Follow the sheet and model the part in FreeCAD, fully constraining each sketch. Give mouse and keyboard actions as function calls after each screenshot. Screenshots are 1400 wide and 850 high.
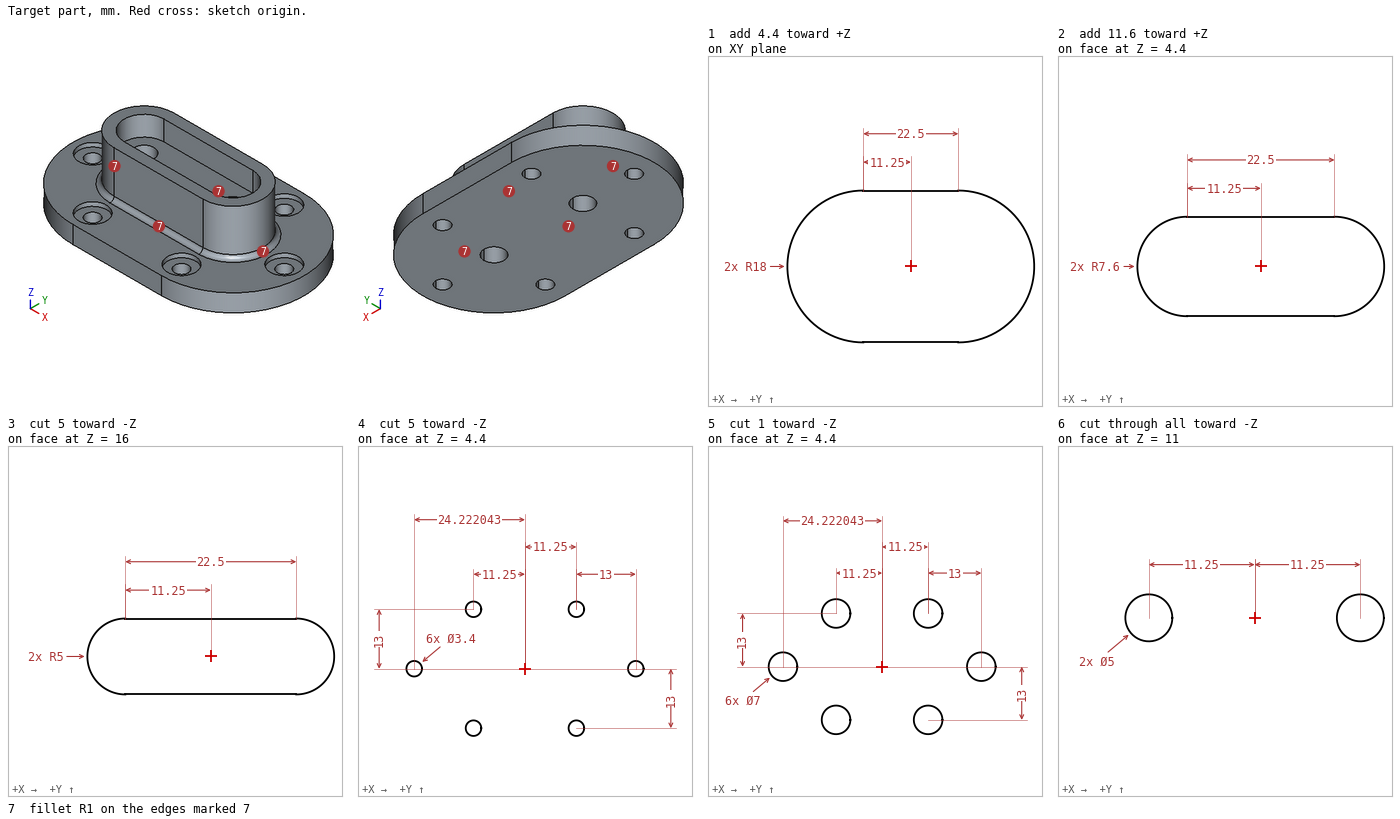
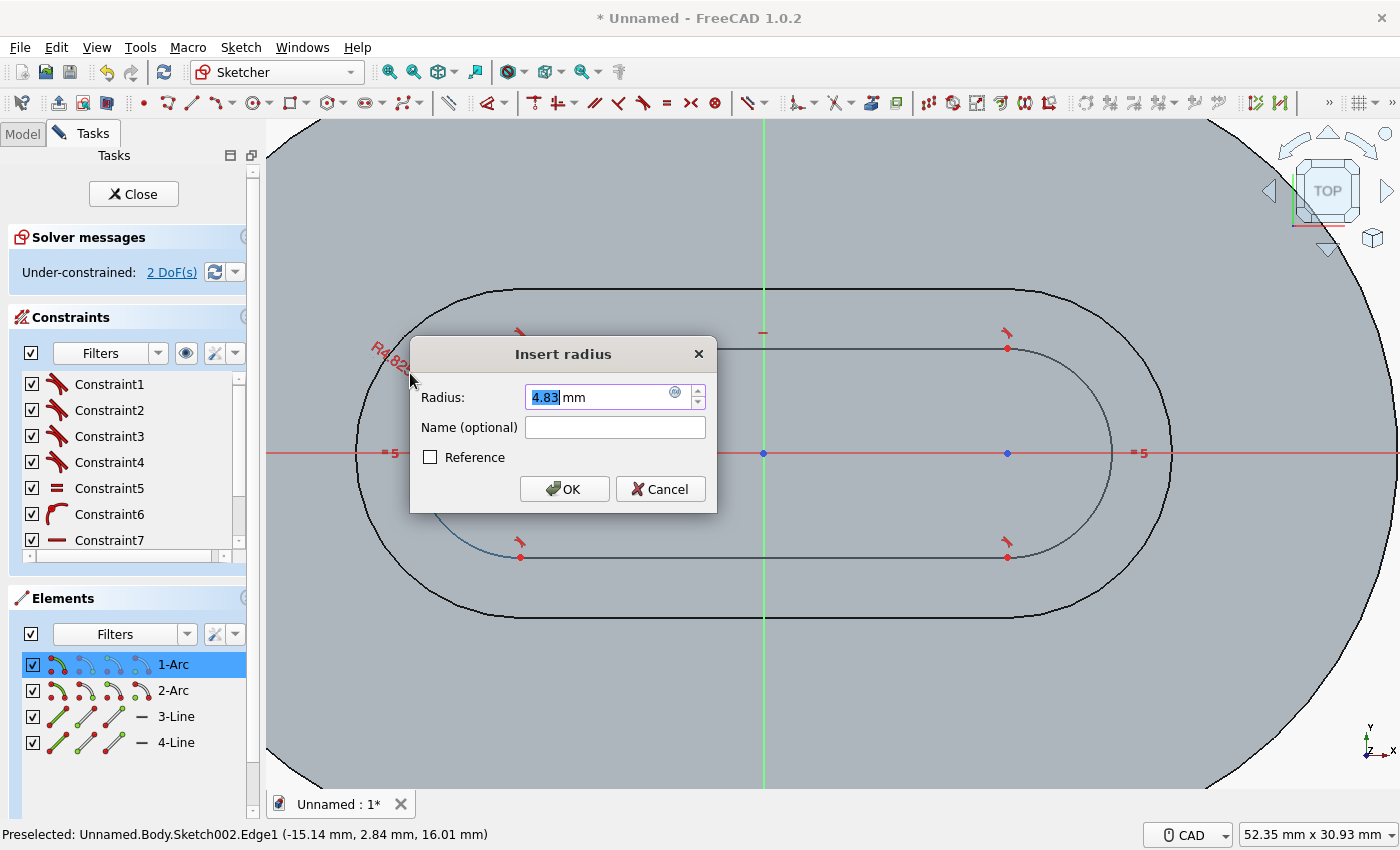
text(5)
key(Return)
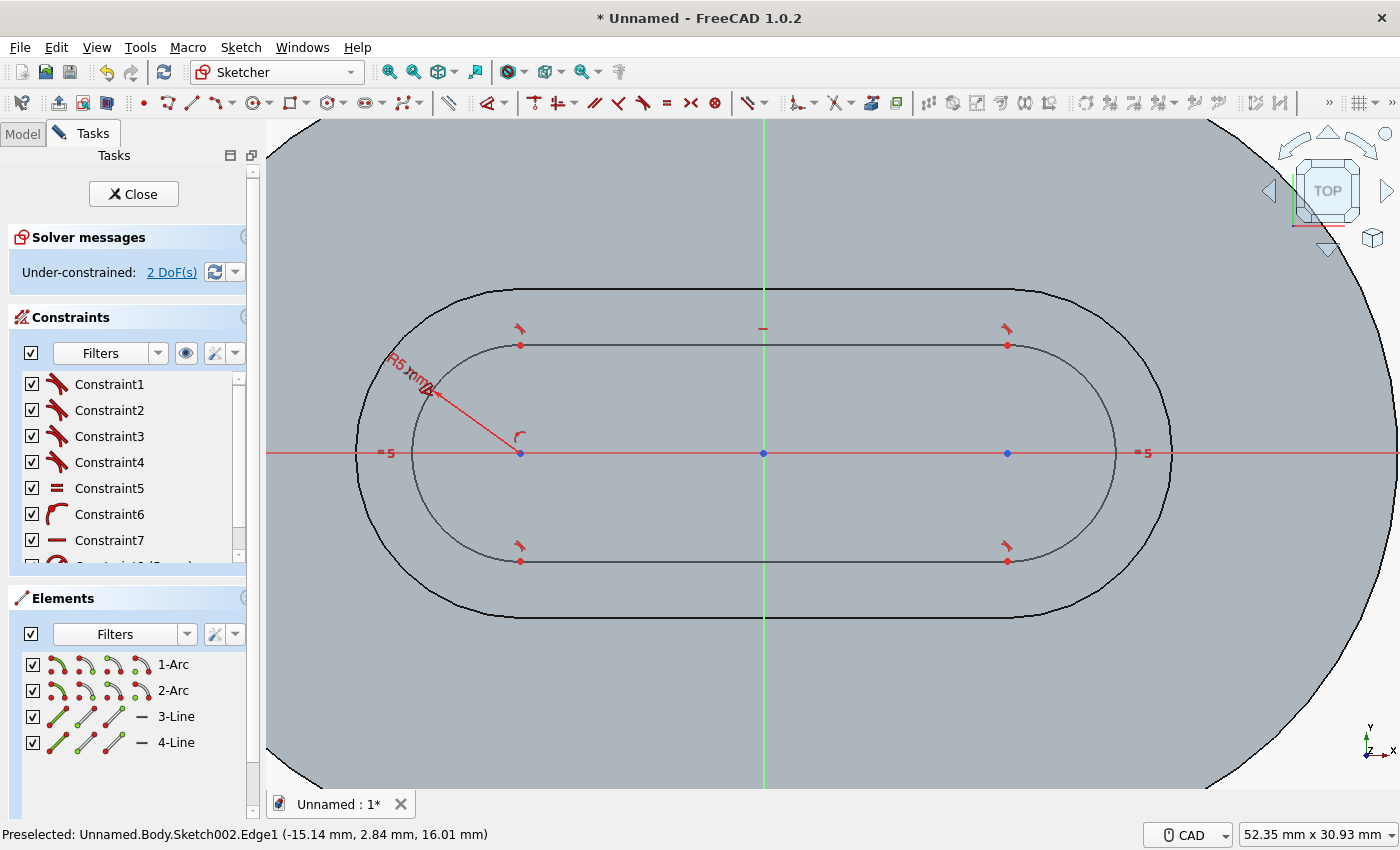
click(667, 345)
click(652, 311)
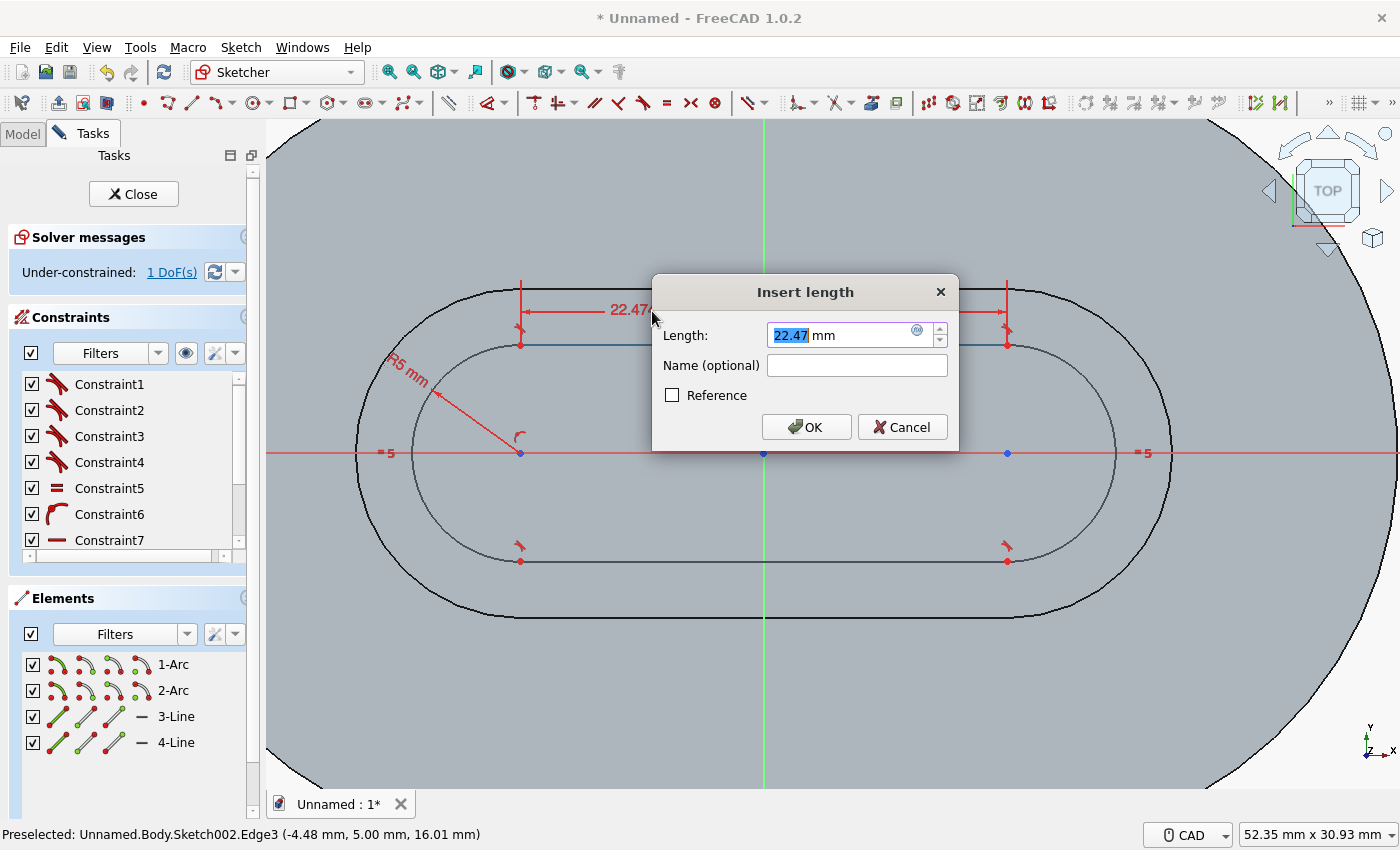
text(22.5)
key(Return)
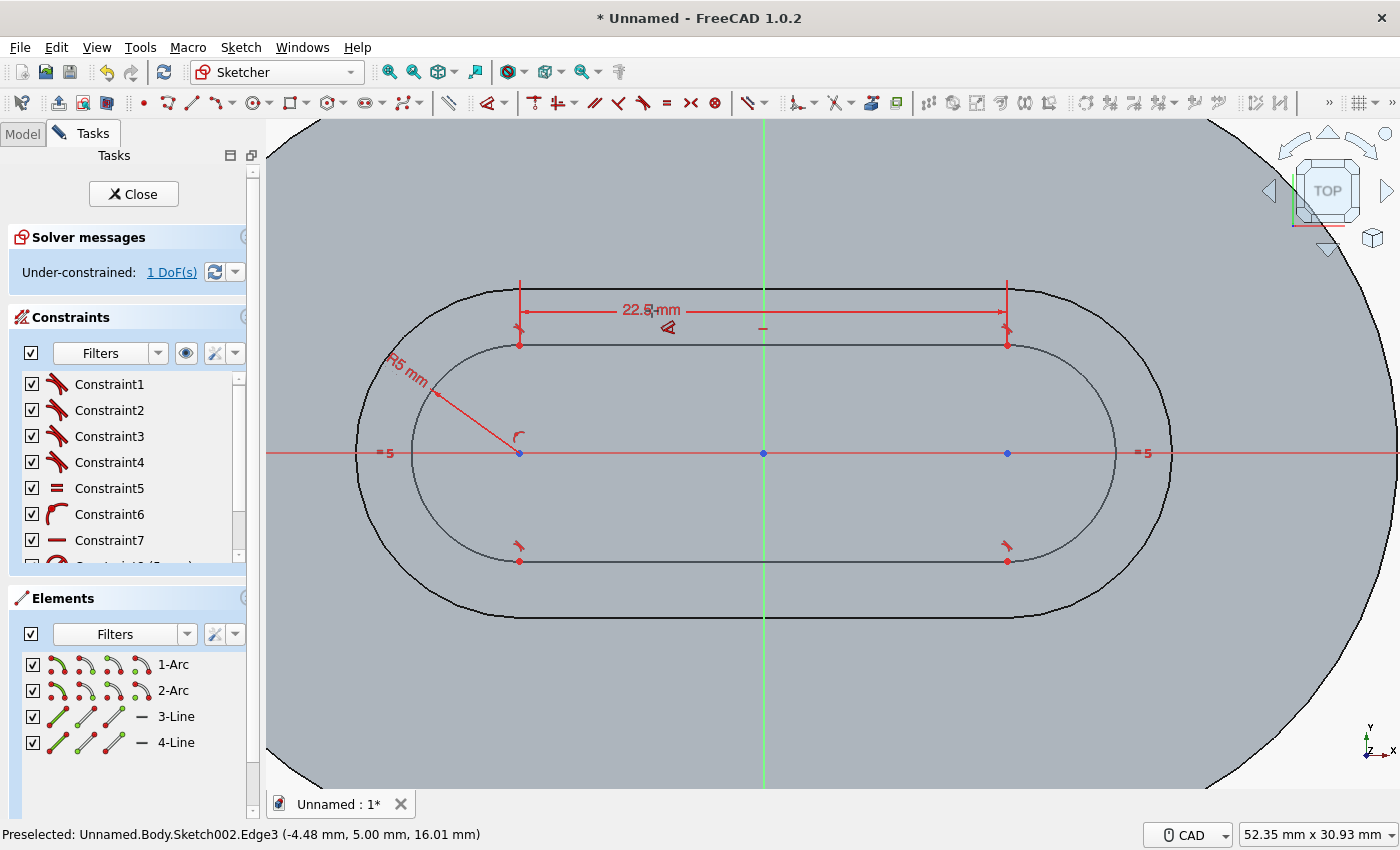
click(520, 345)
click(557, 311)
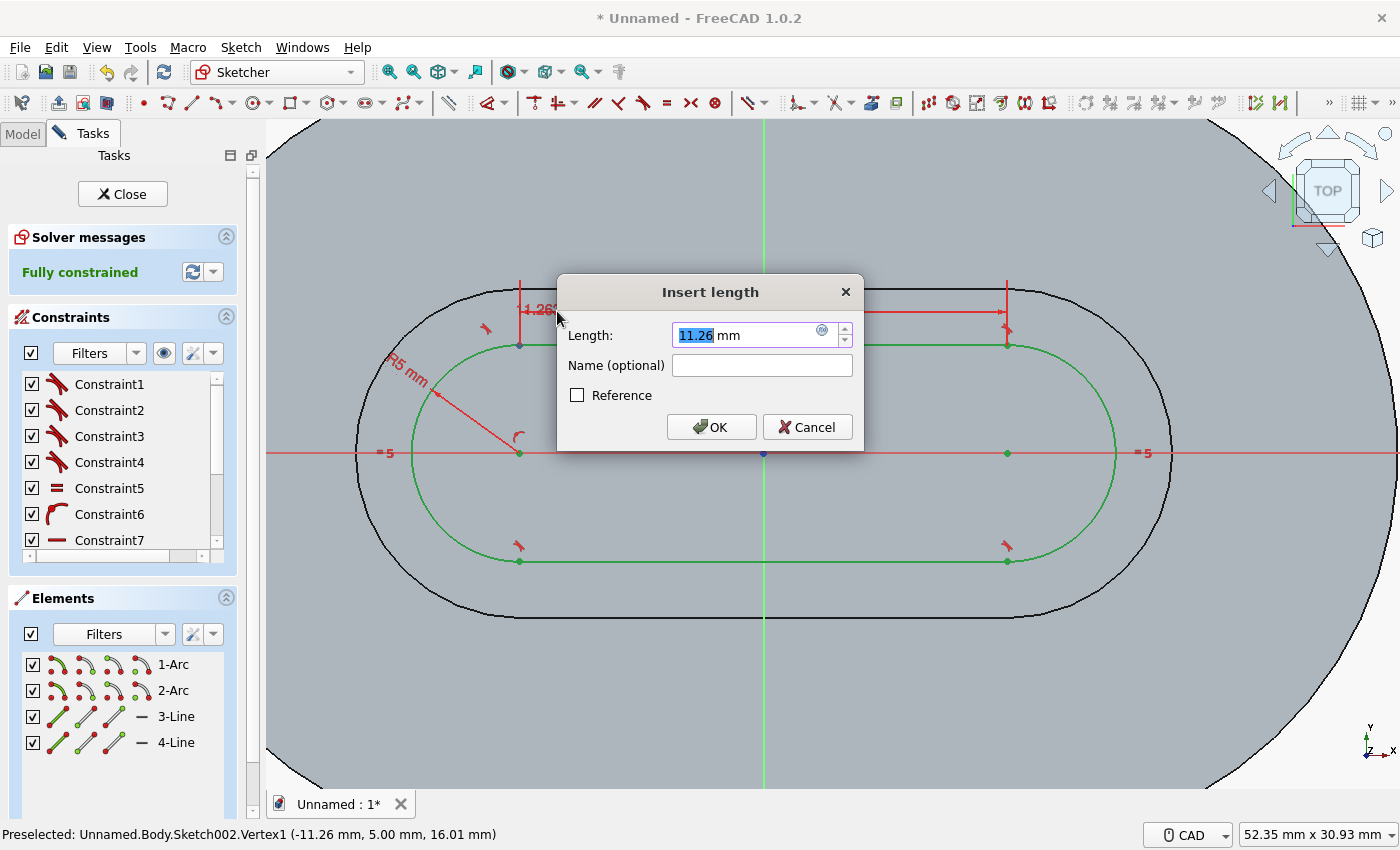
text(11.25)
key(Return)
key(Escape)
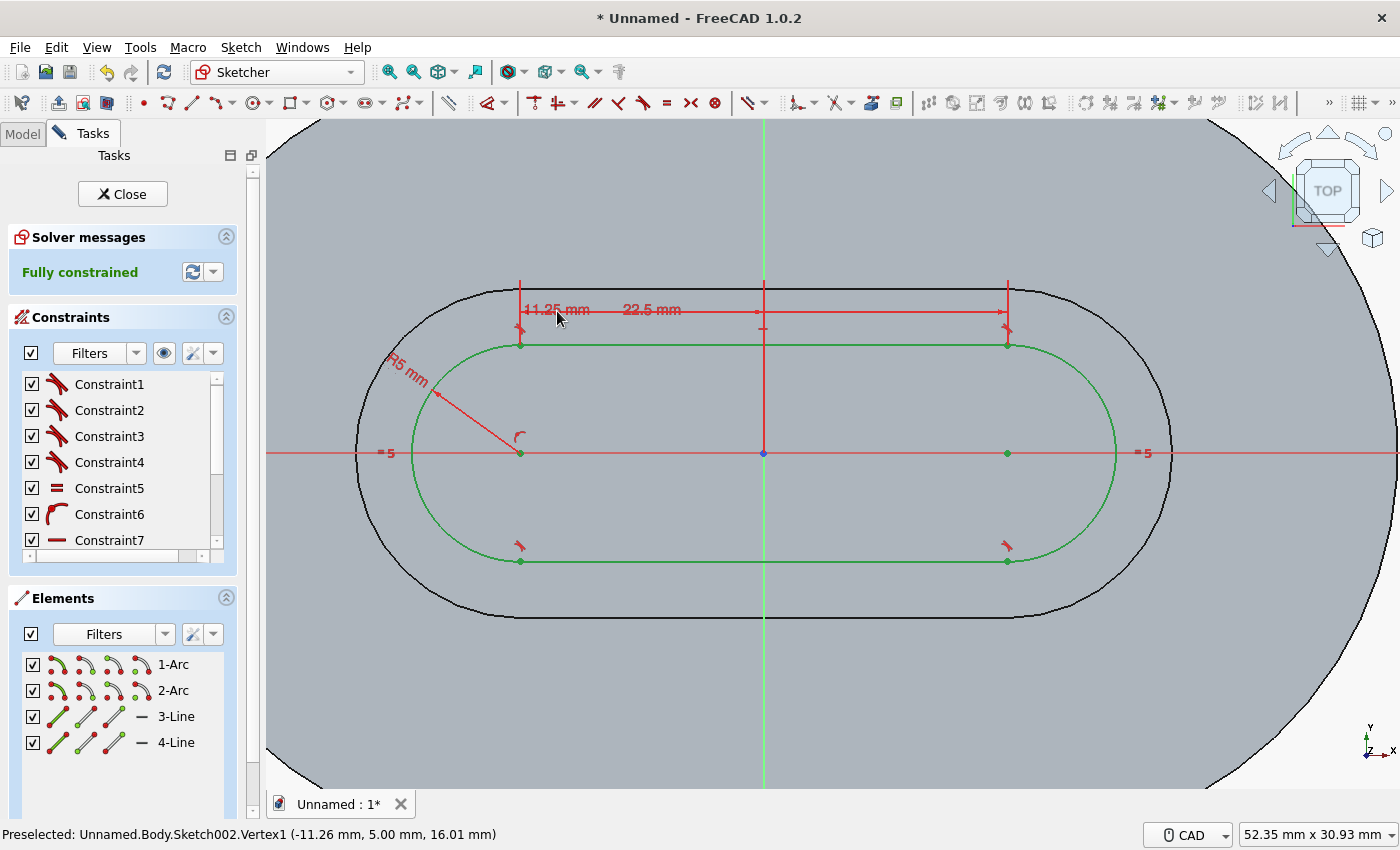
click(123, 194)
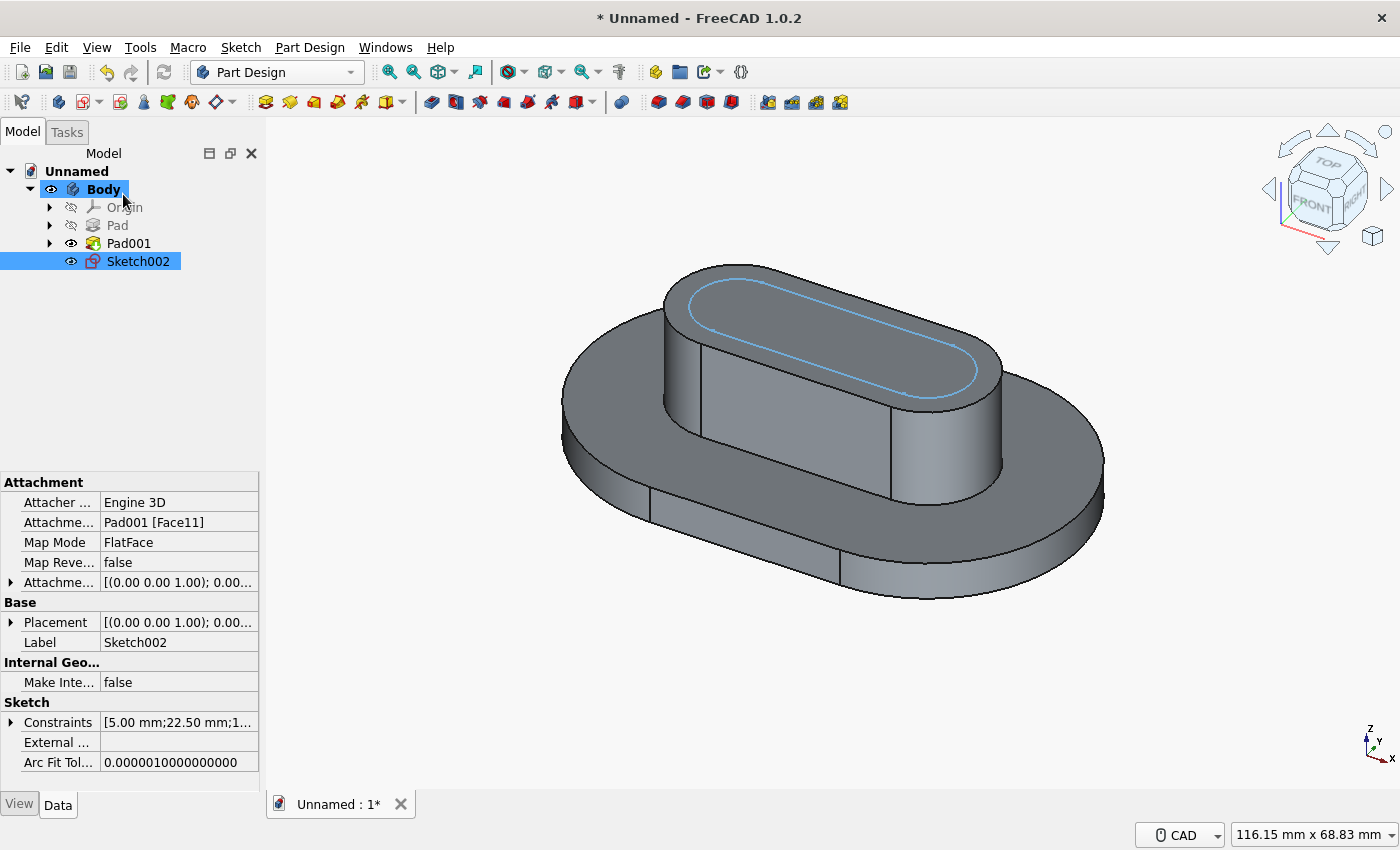
click(432, 102)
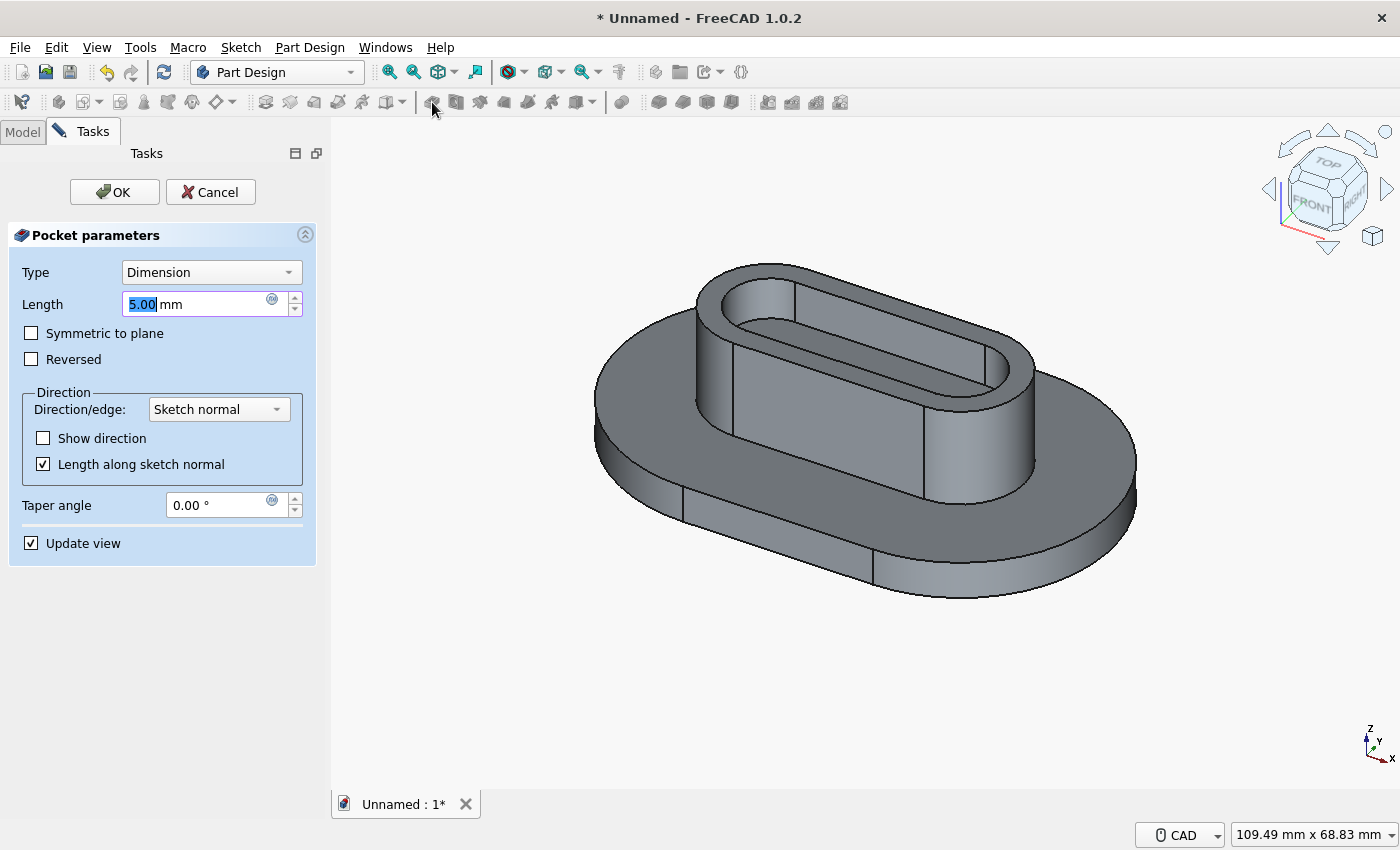
text(5)
key(Tab)